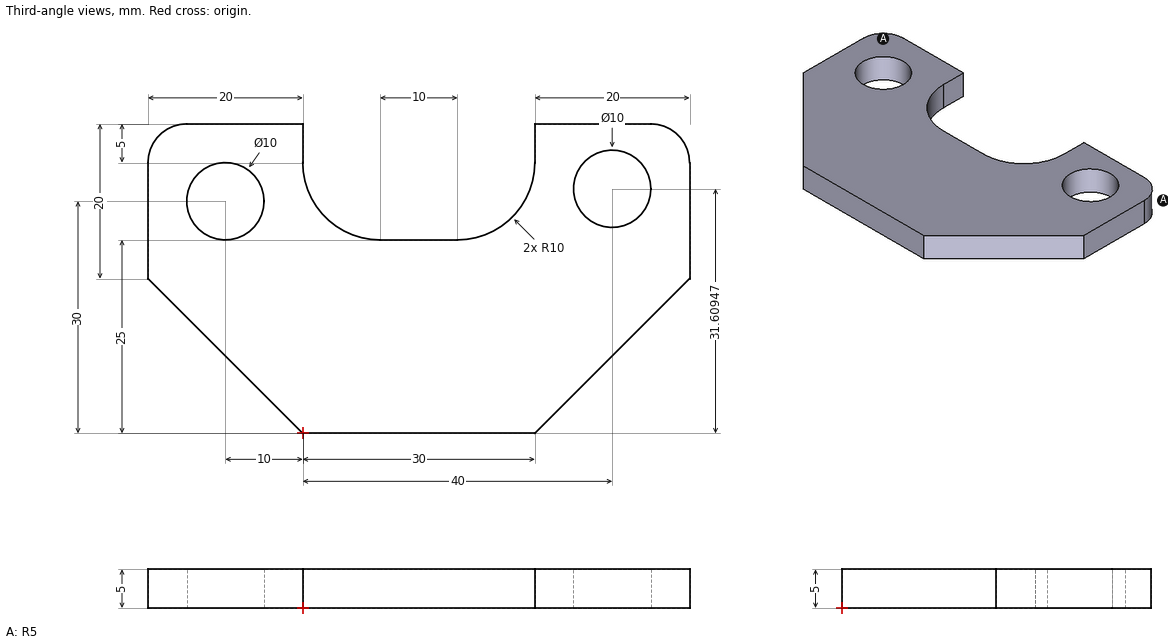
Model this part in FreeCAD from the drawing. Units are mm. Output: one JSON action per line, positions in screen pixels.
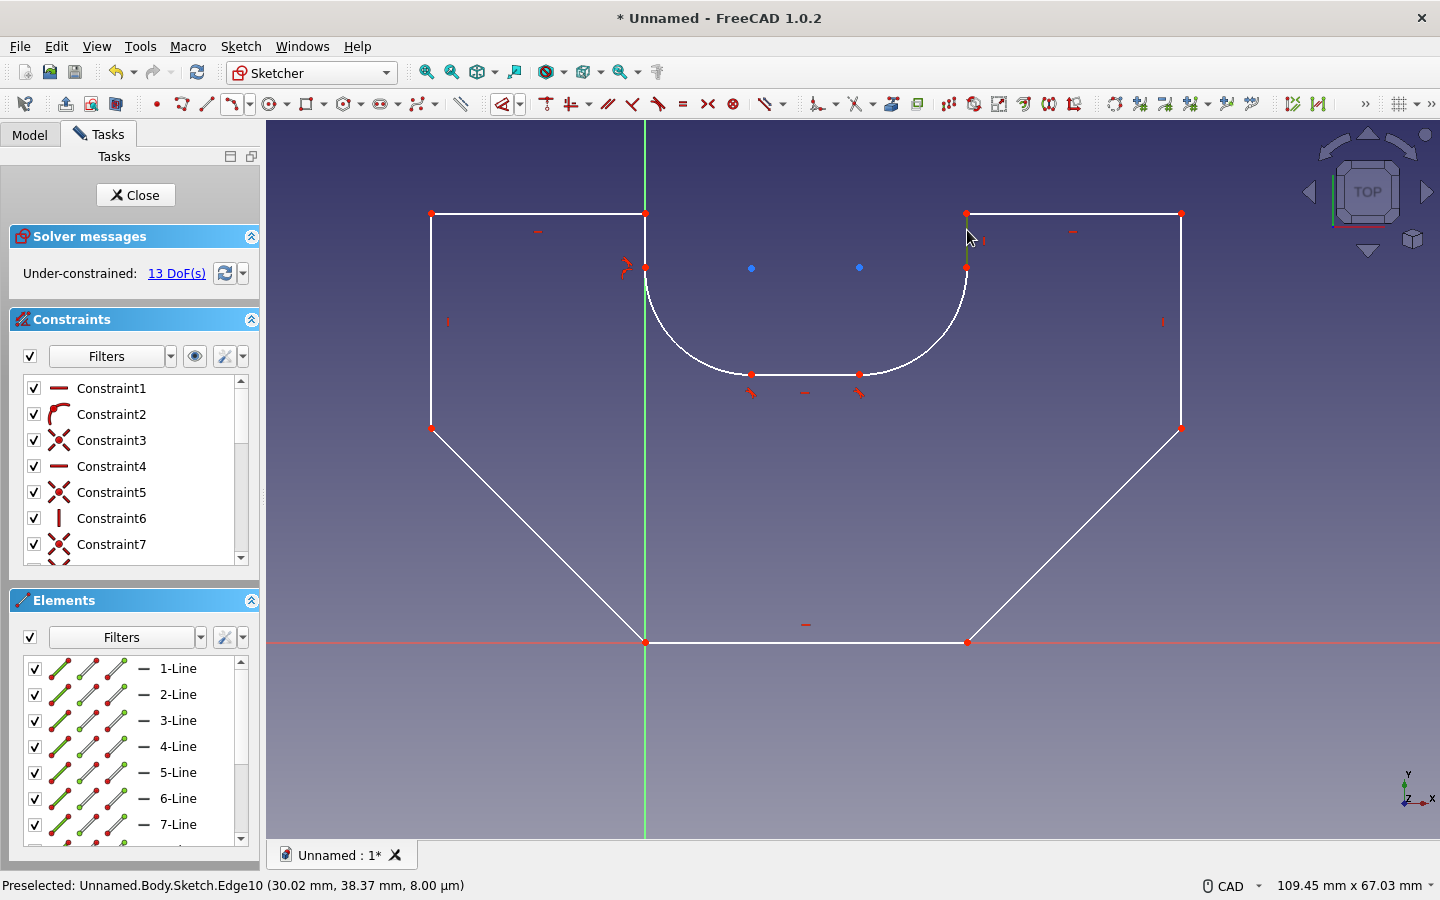
{"action": "left_click", "coordinate": [908, 363]}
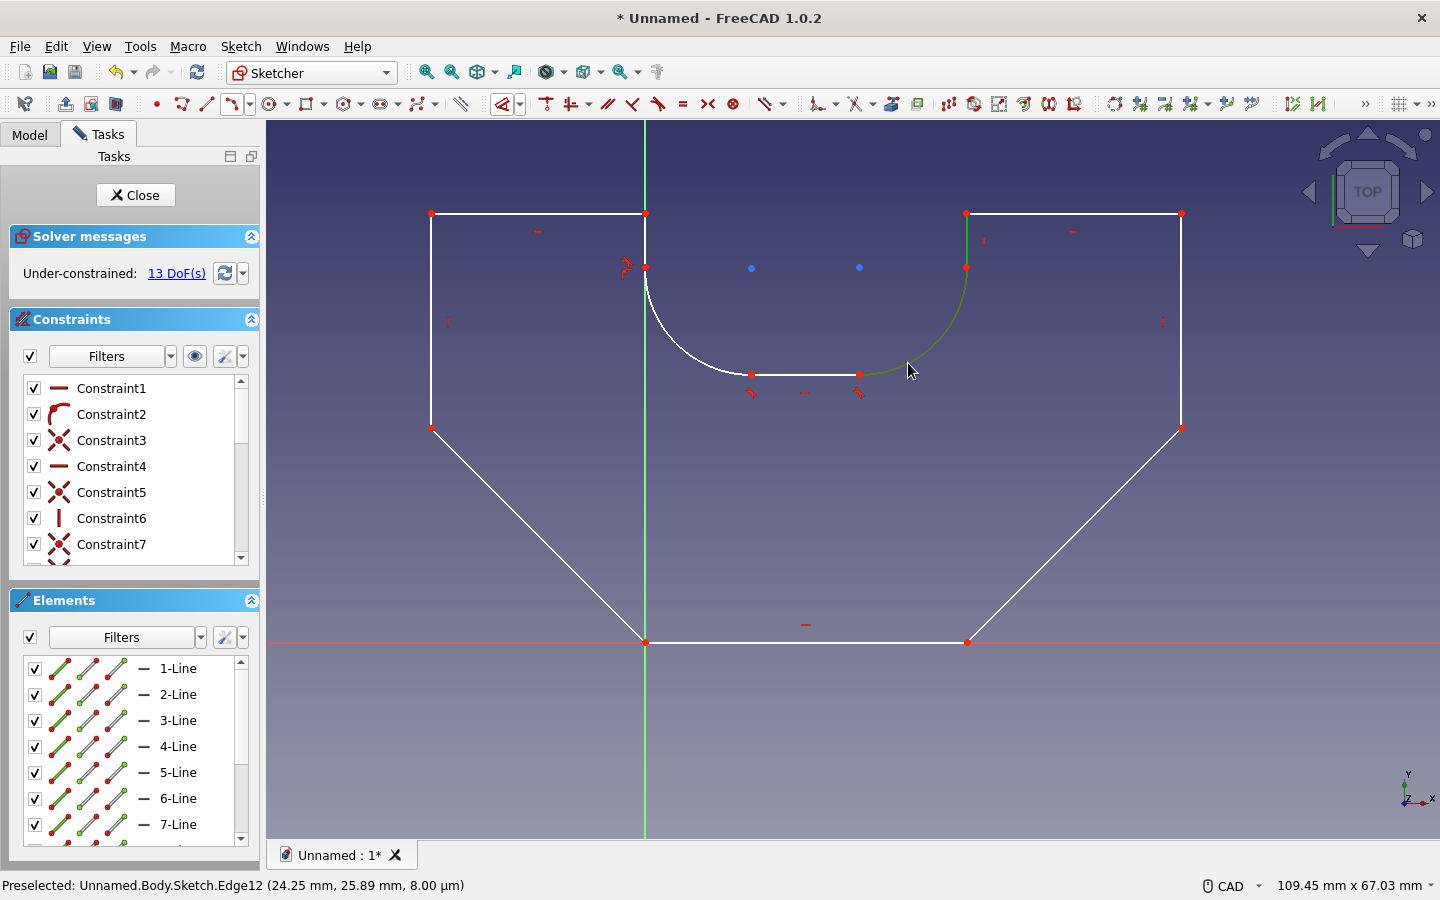
{"action": "left_click", "coordinate": [658, 104]}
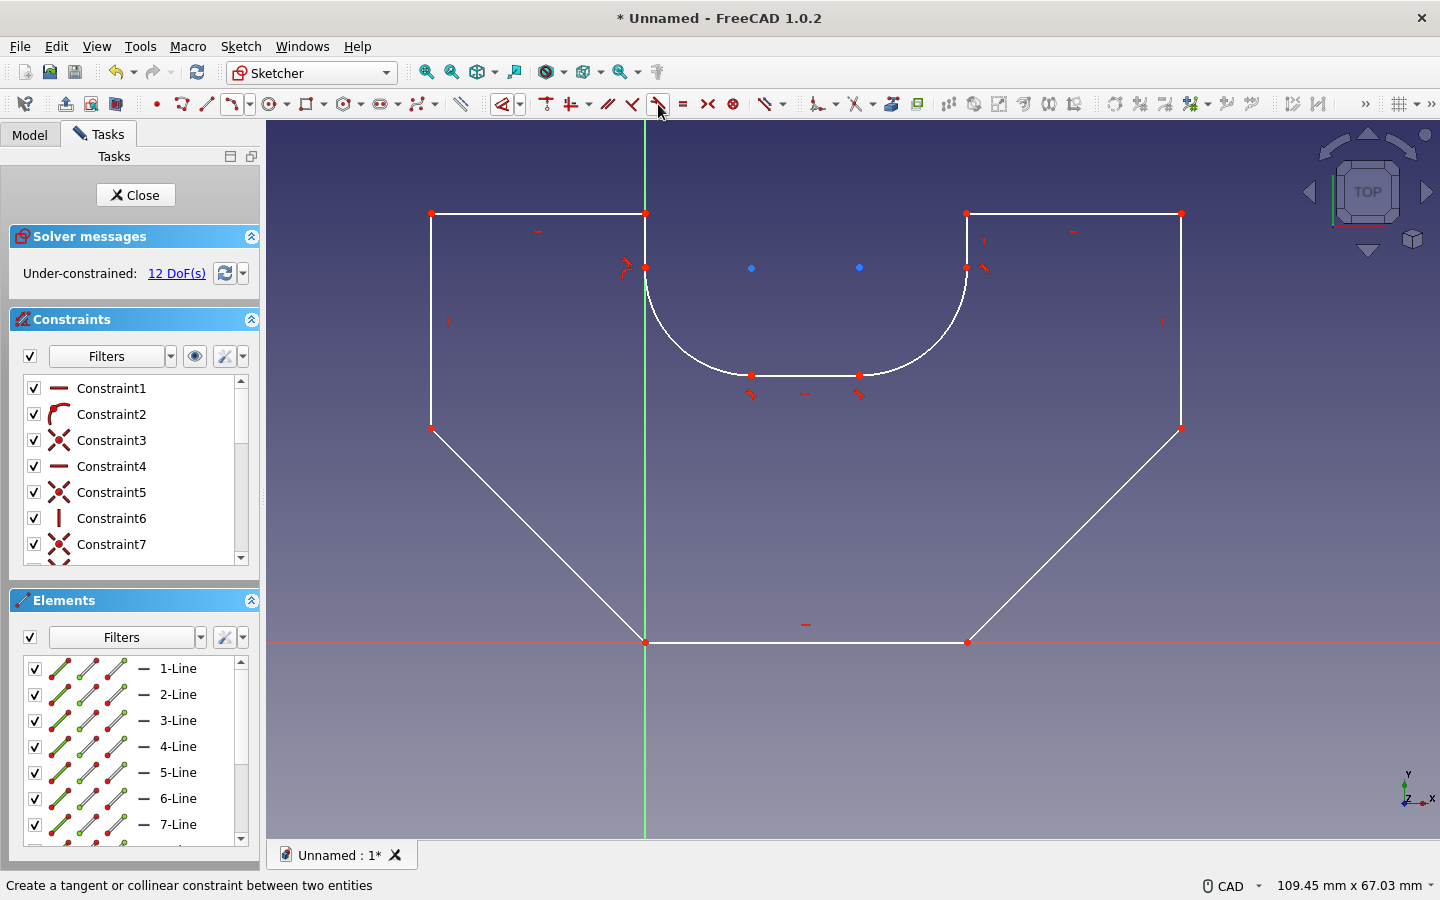
{"action": "left_click", "coordinate": [645, 252]}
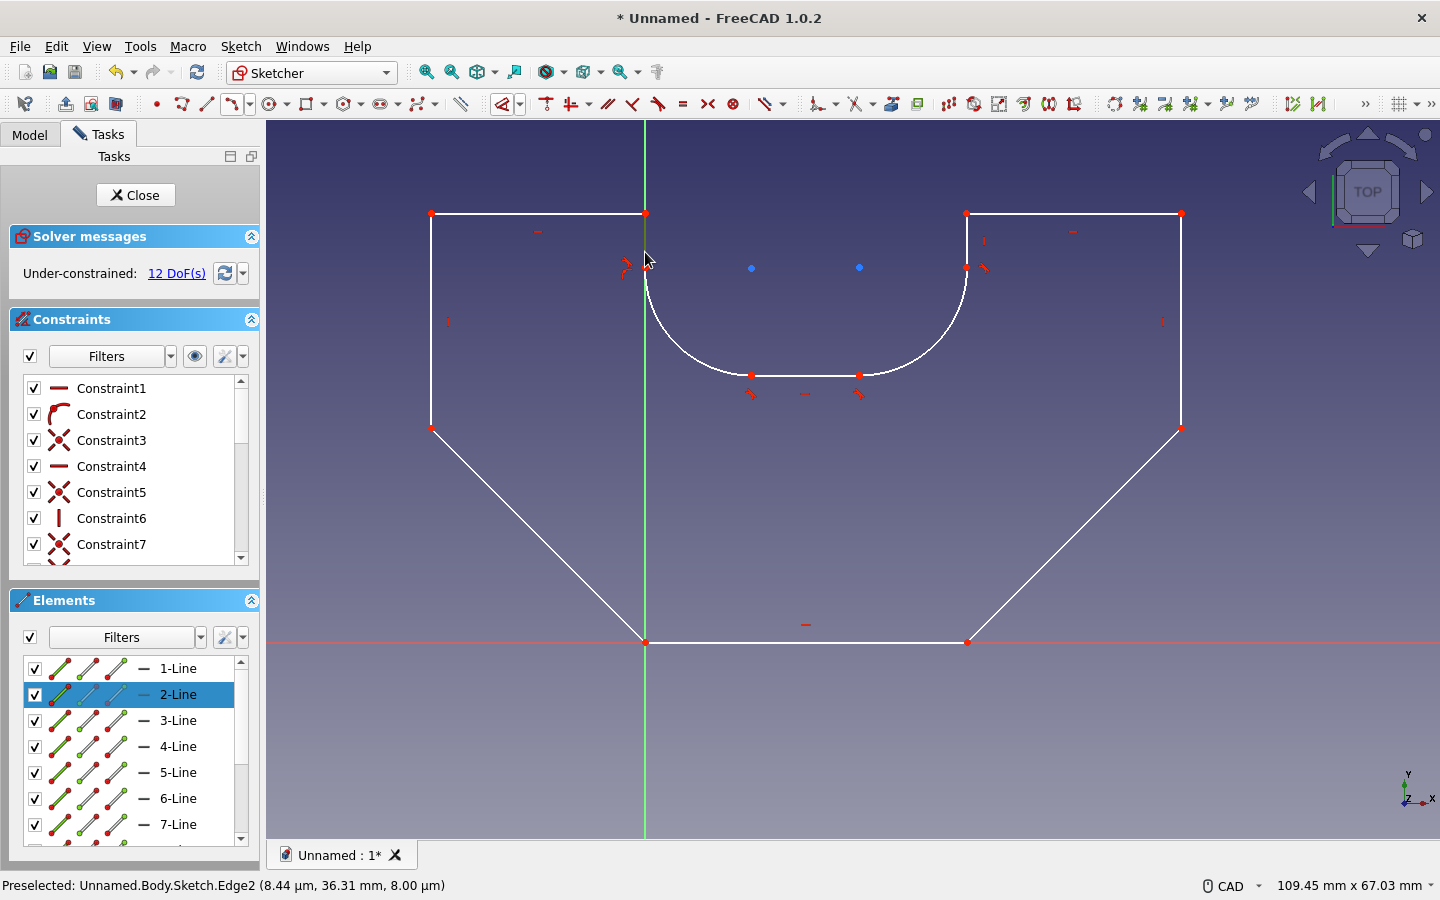
{"action": "left_click", "coordinate": [588, 104]}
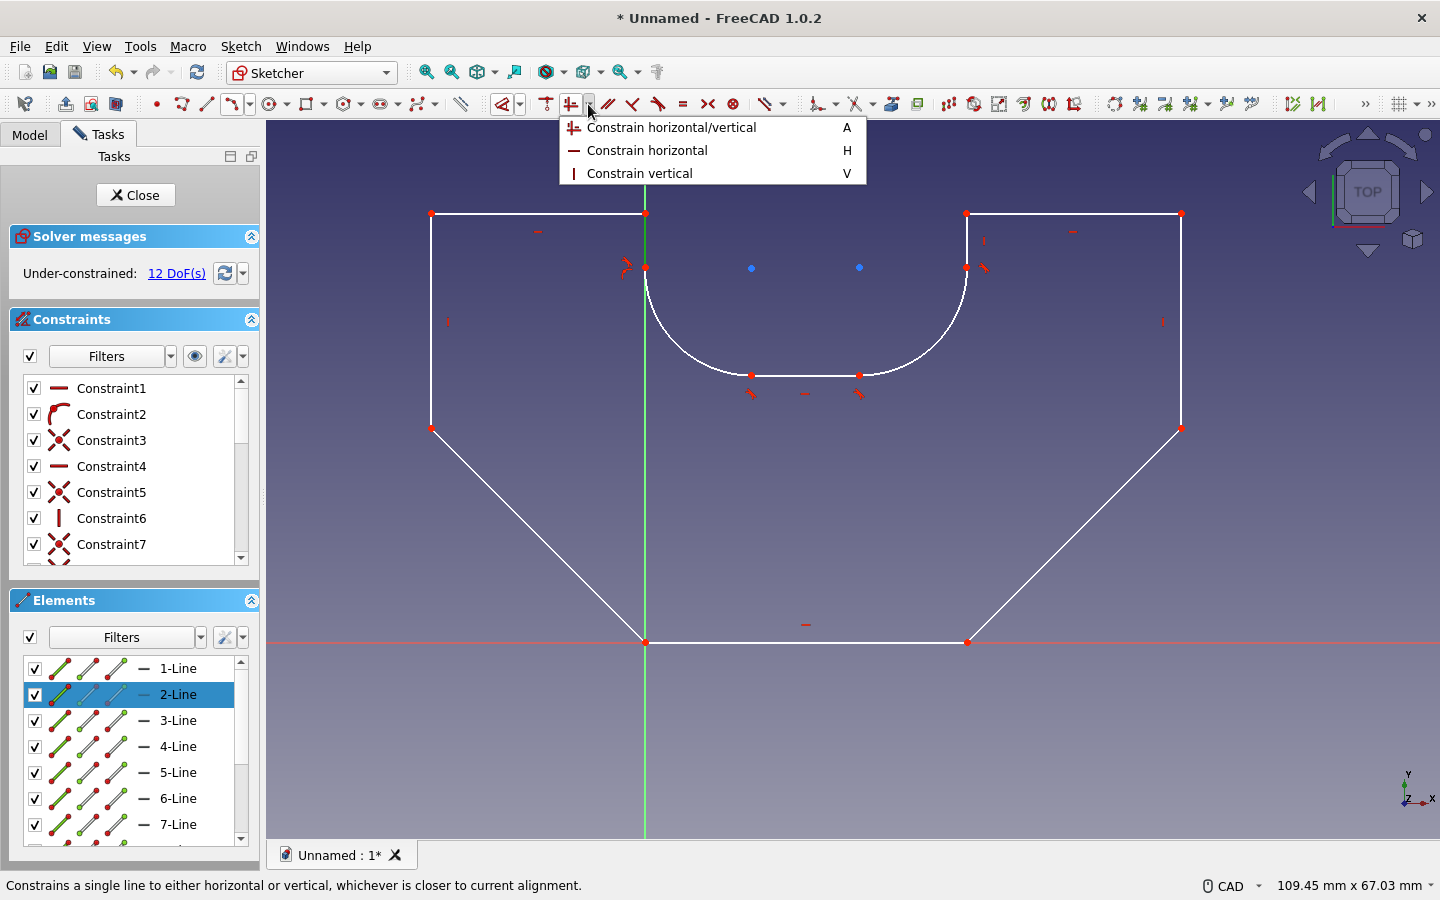
{"action": "left_click", "coordinate": [713, 174]}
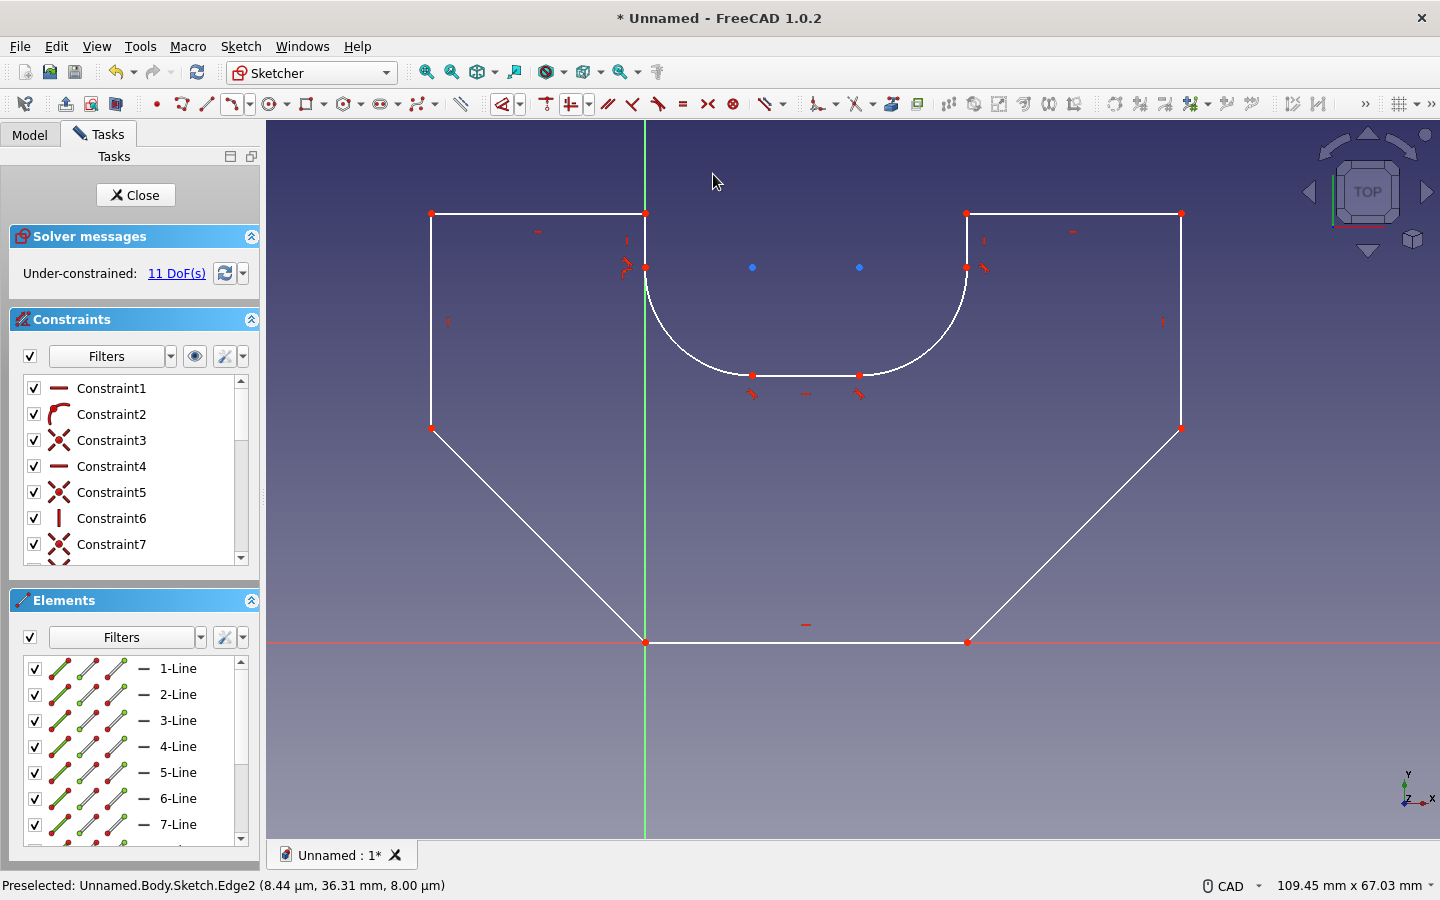
{"action": "left_click", "coordinate": [657, 317]}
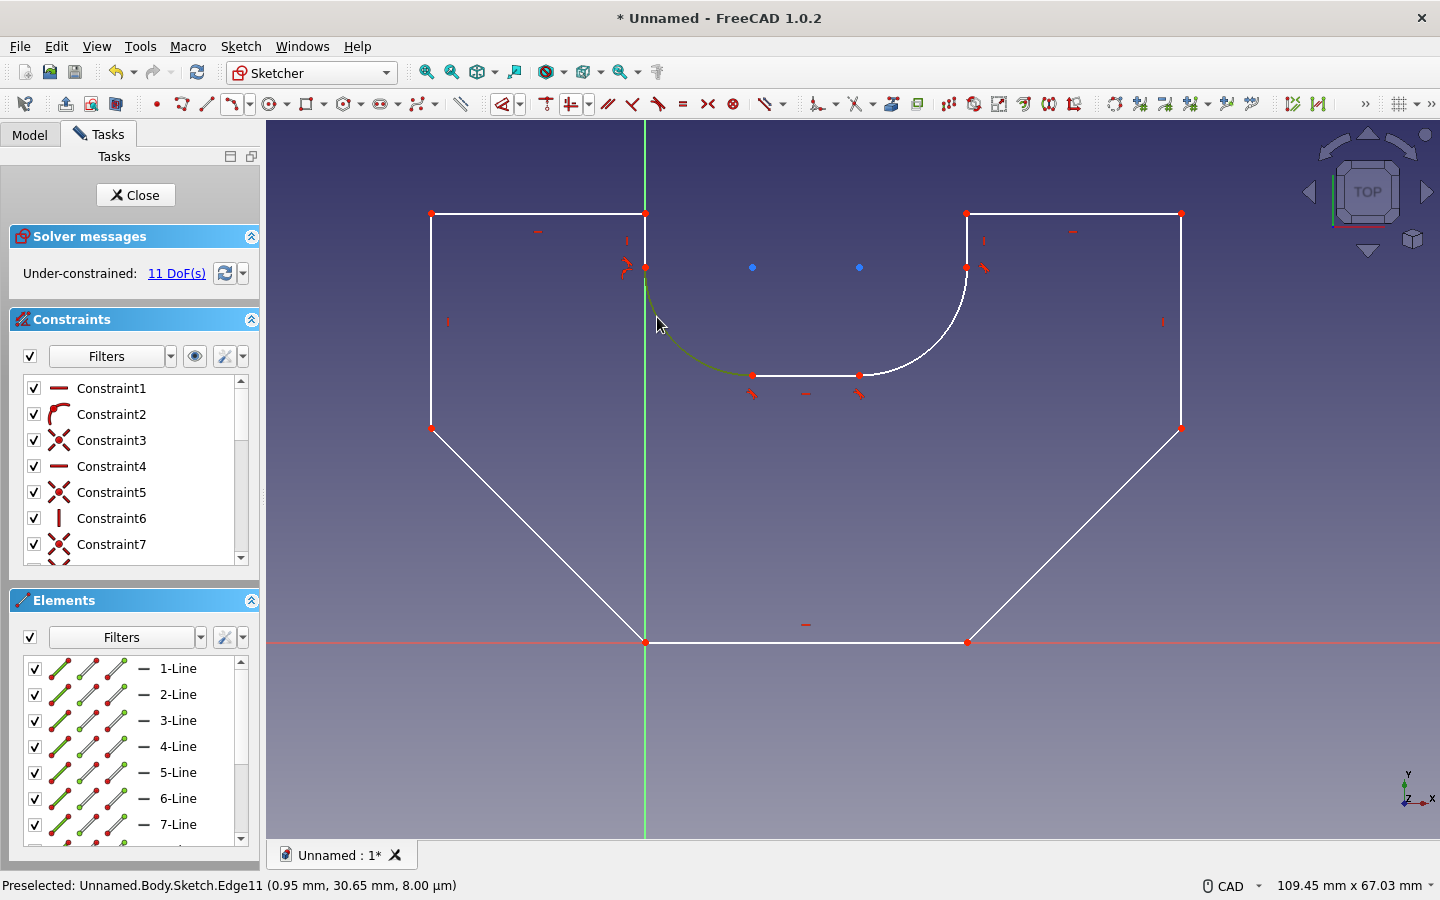
{"action": "left_click", "coordinate": [908, 364]}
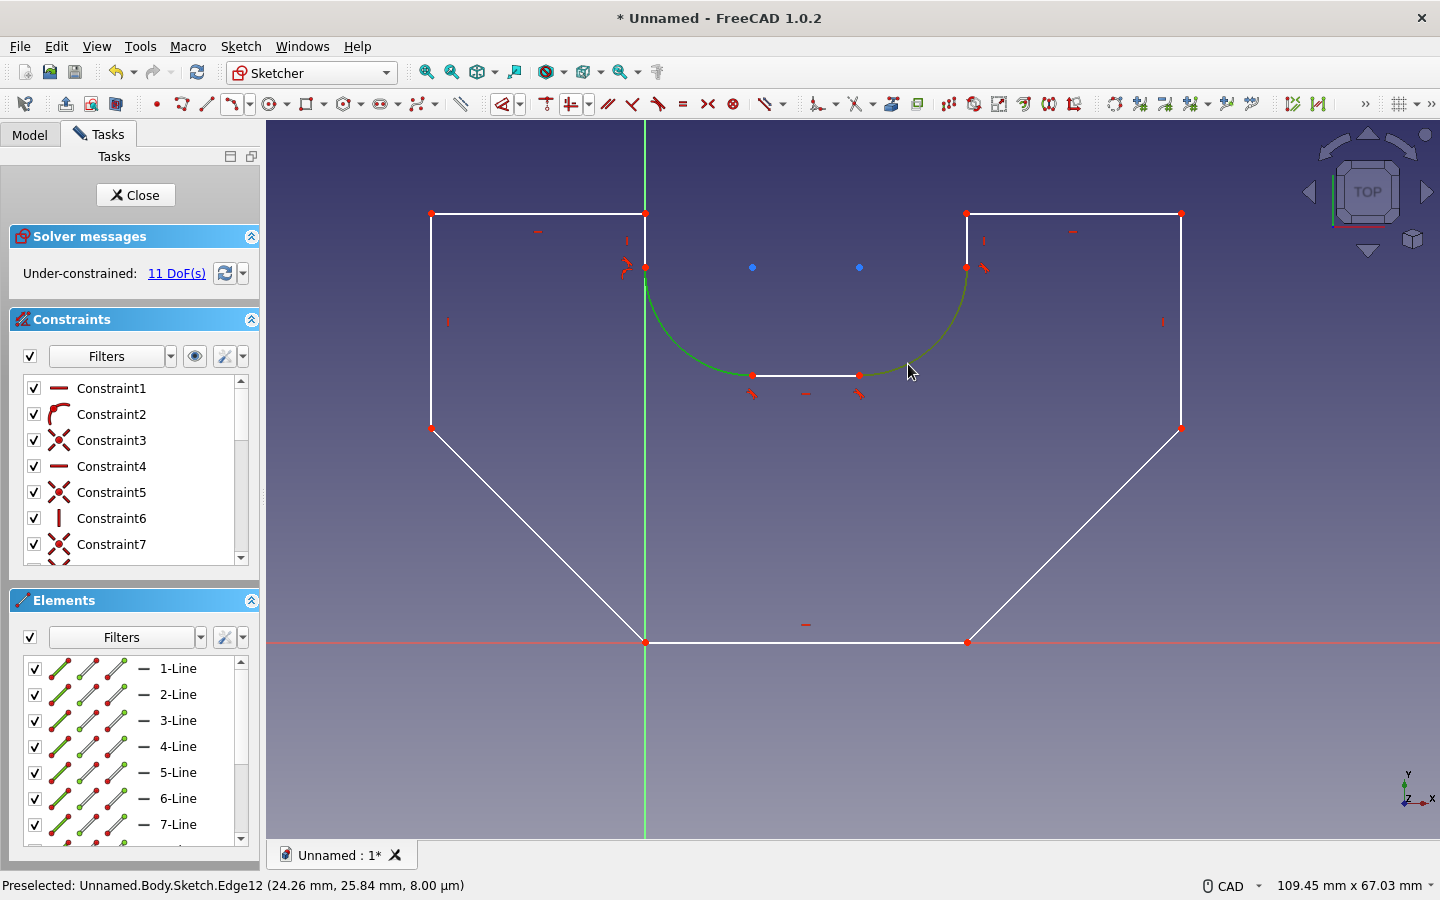
{"action": "left_click", "coordinate": [683, 104]}